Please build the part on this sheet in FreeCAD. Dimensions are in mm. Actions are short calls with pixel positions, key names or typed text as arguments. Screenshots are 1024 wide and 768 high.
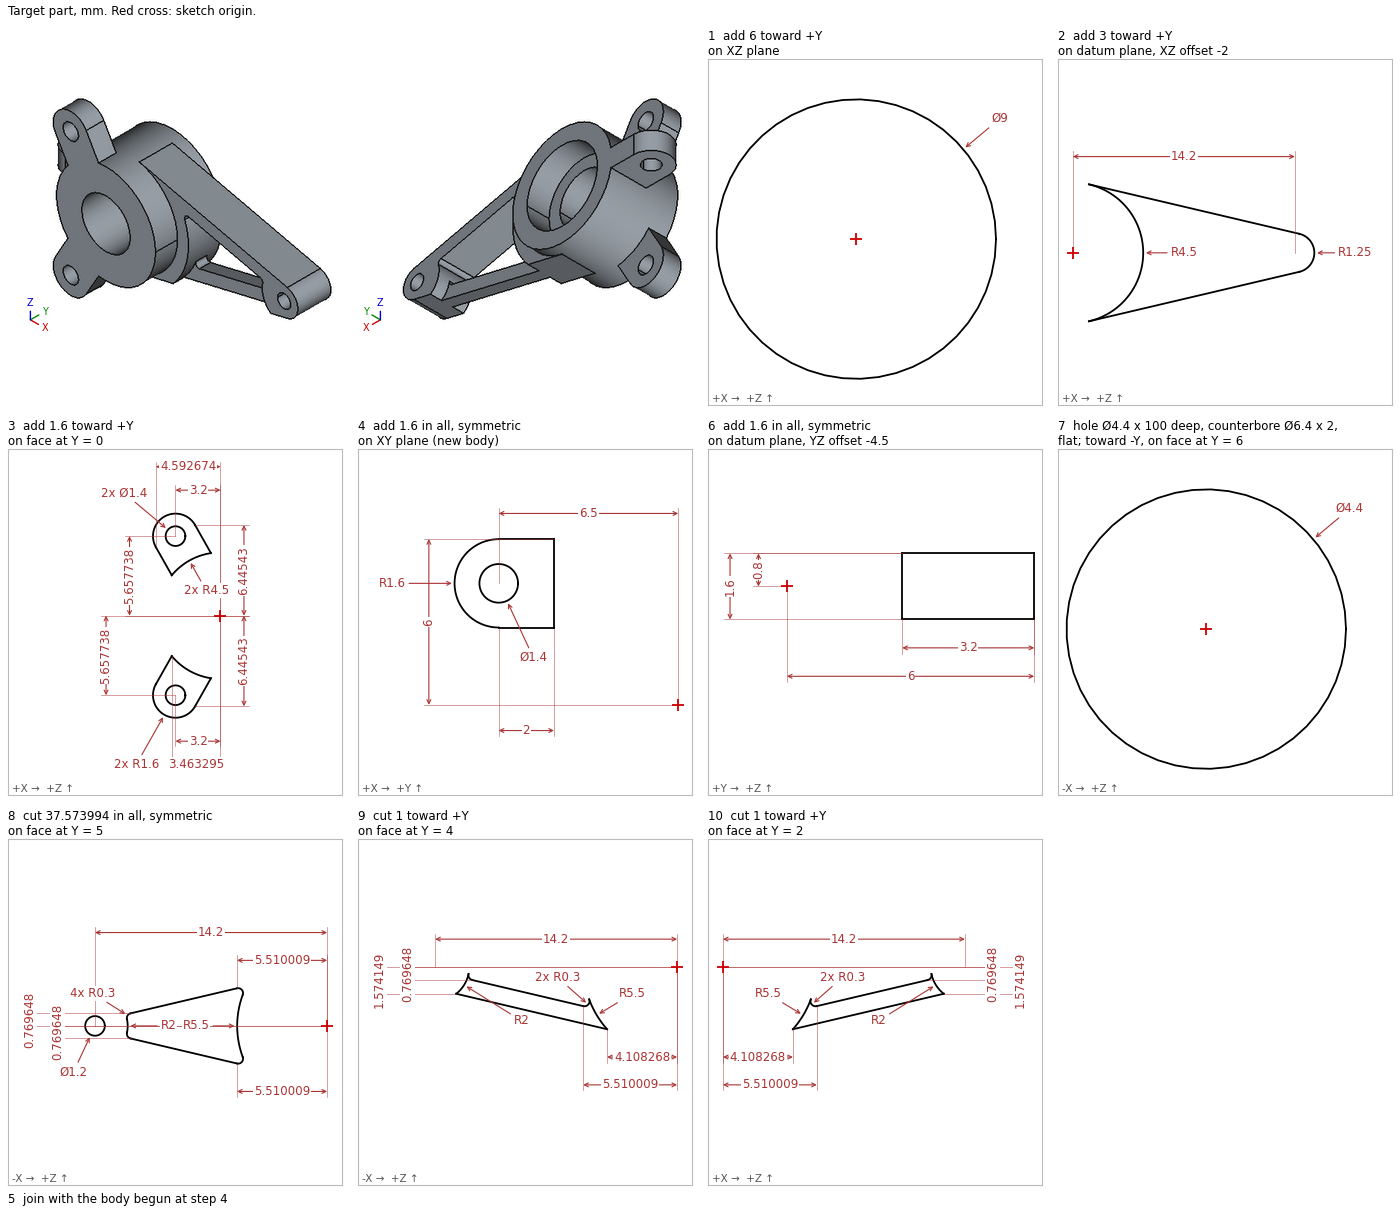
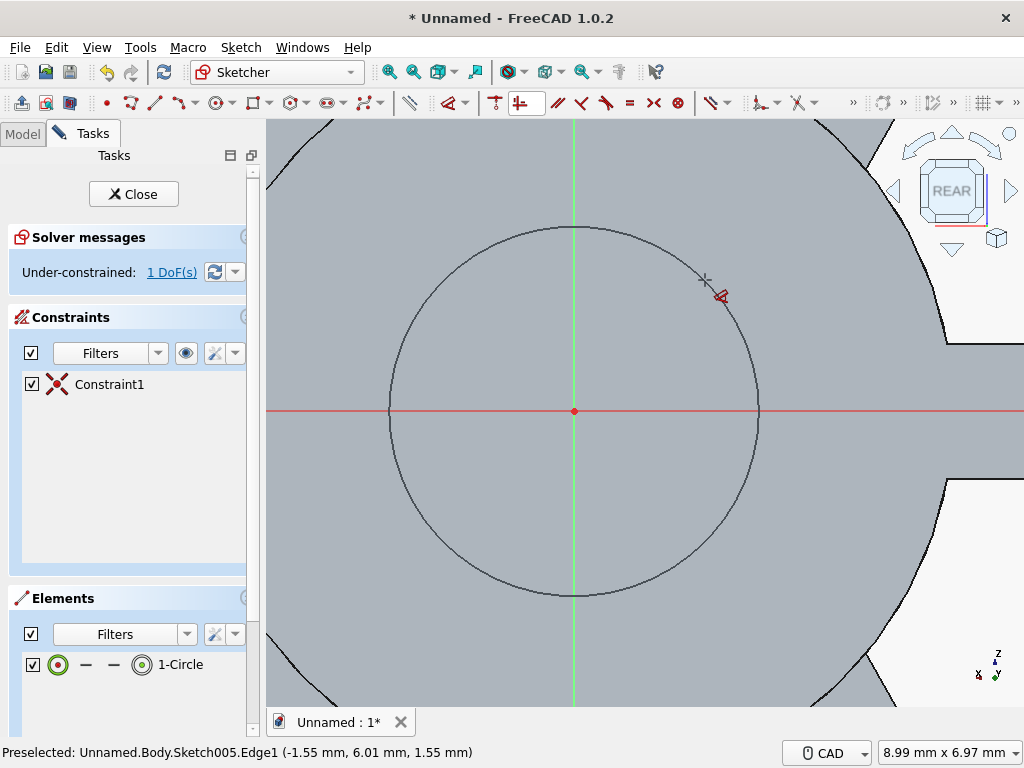
click(704, 280)
click(726, 257)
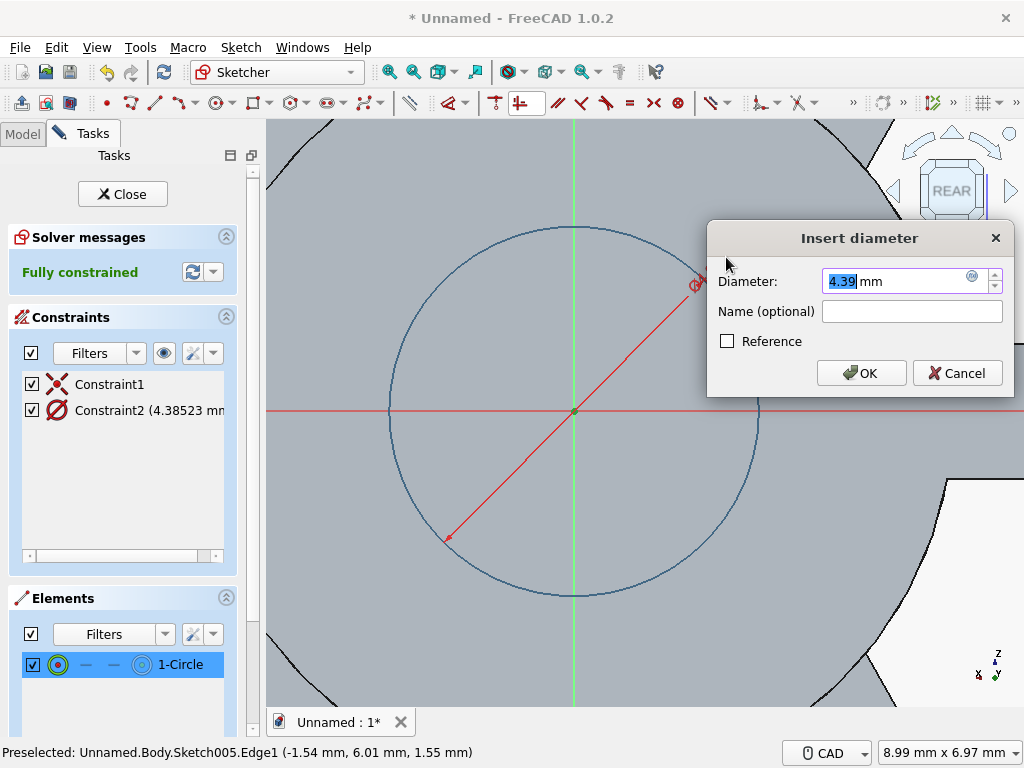
text(4.4)
key(Return)
key(Escape)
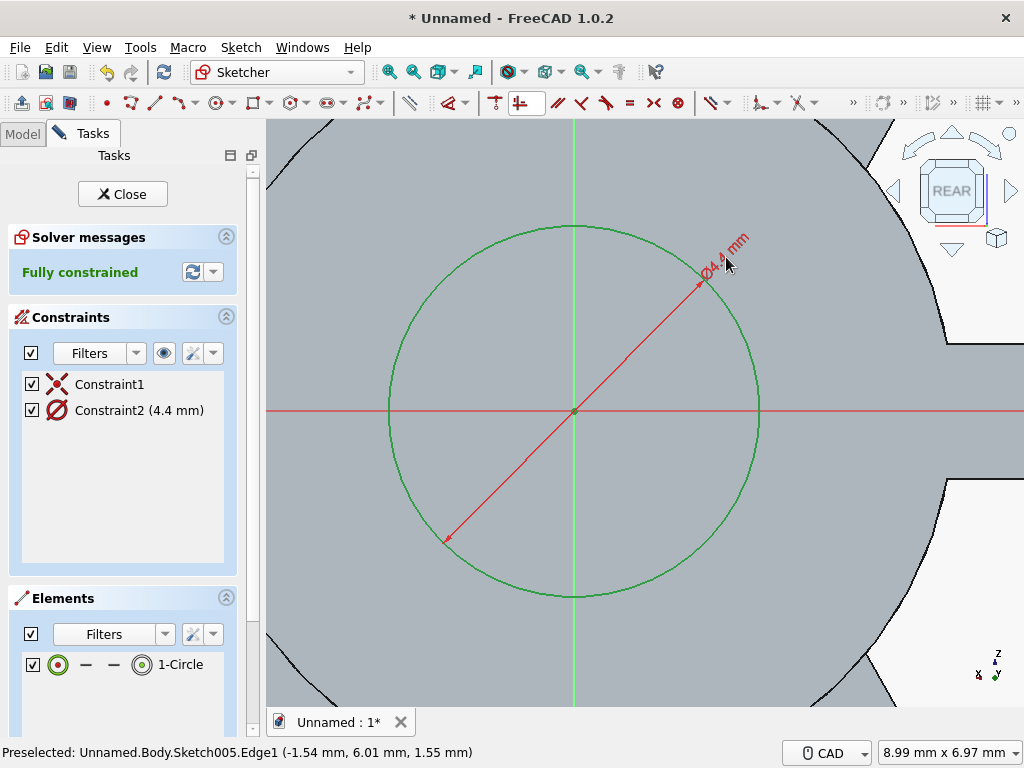
click(123, 194)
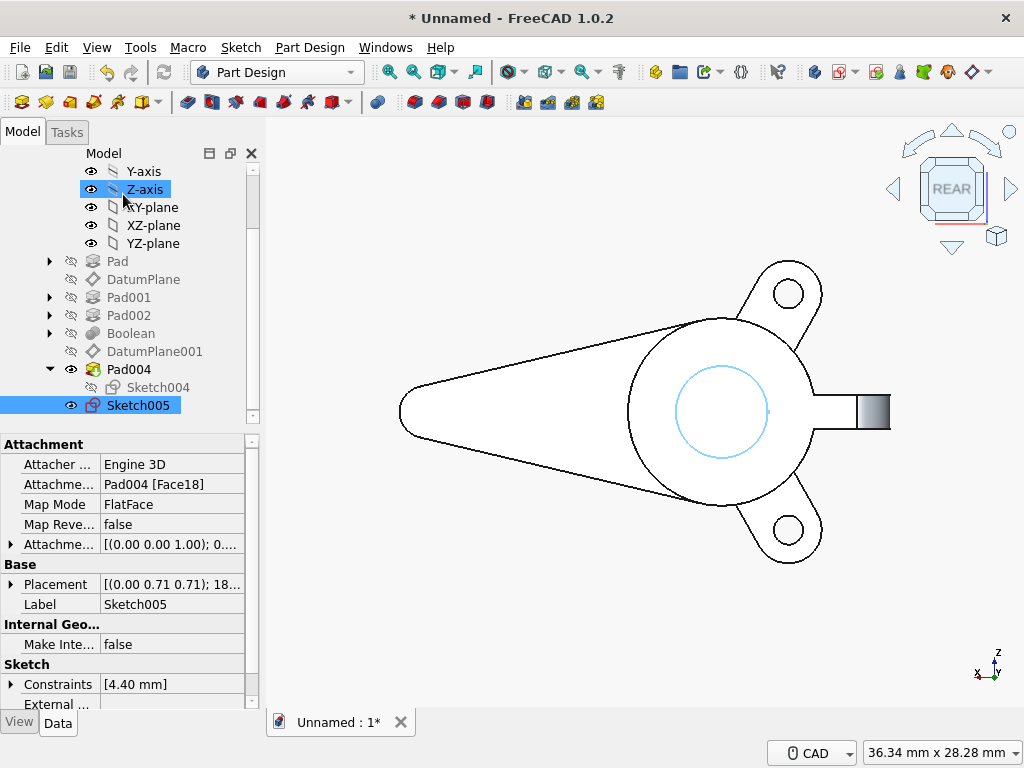
click(212, 102)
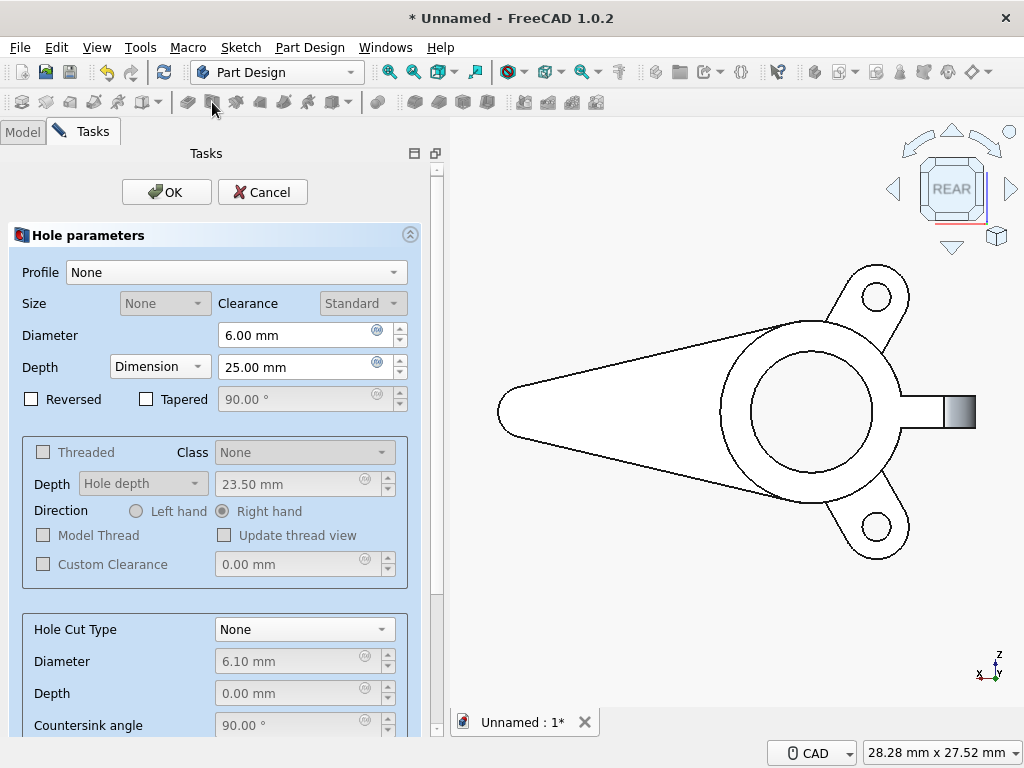
triple_click(305, 335)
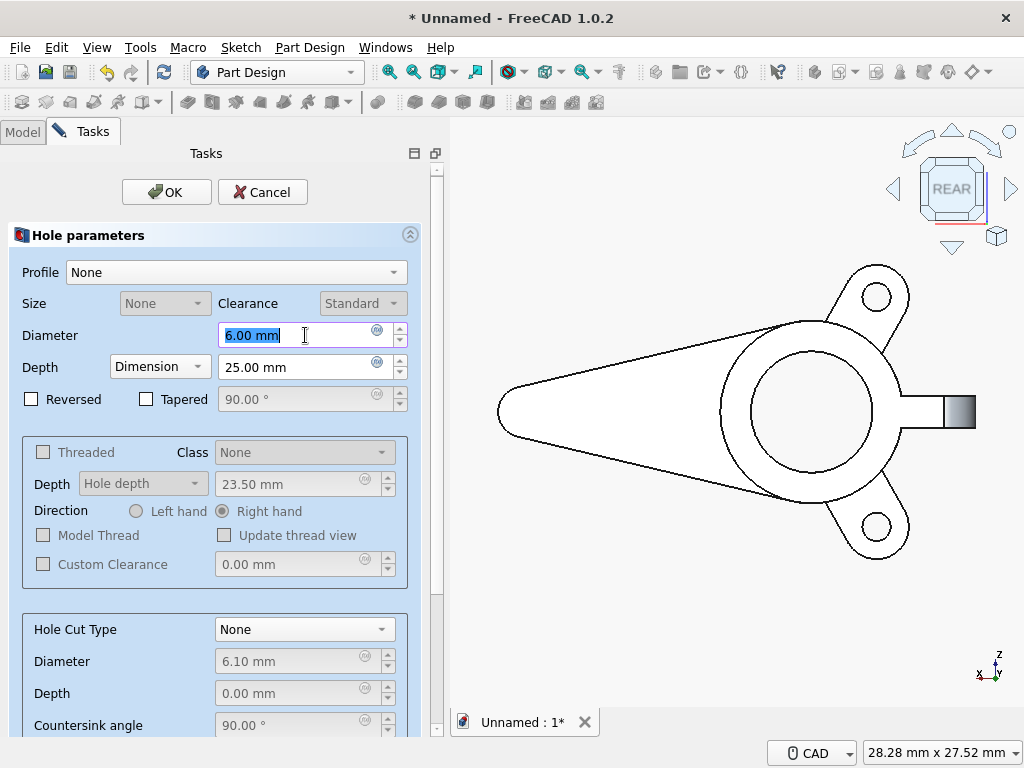
text(4.4)
key(Tab)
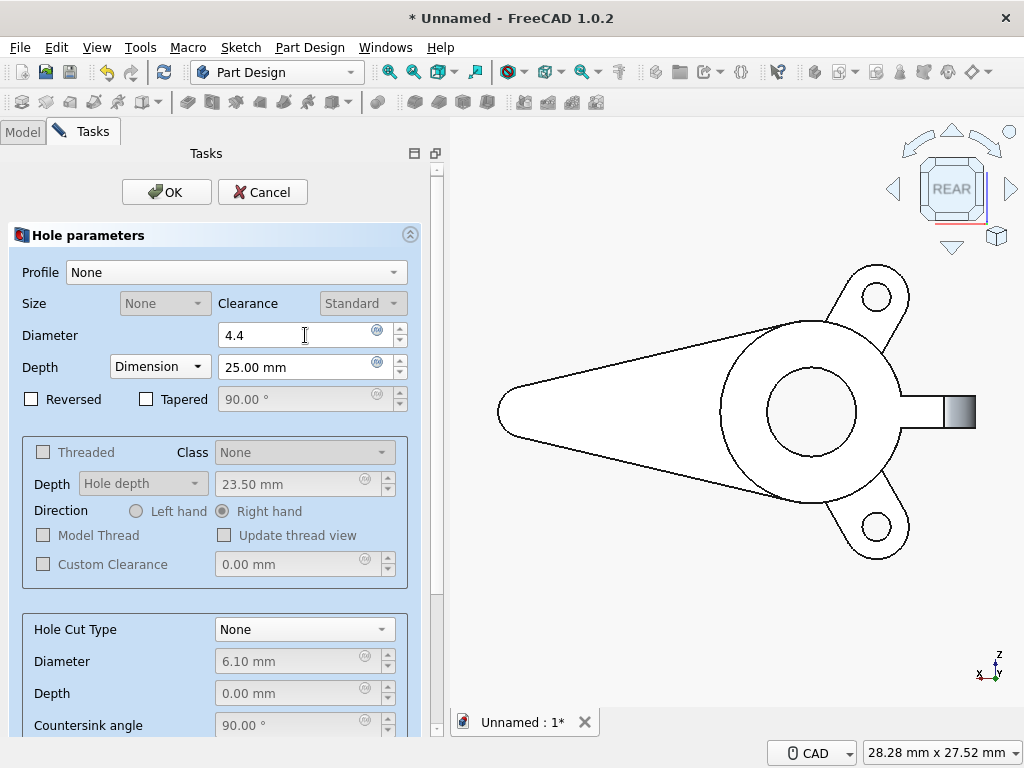
triple_click(305, 367)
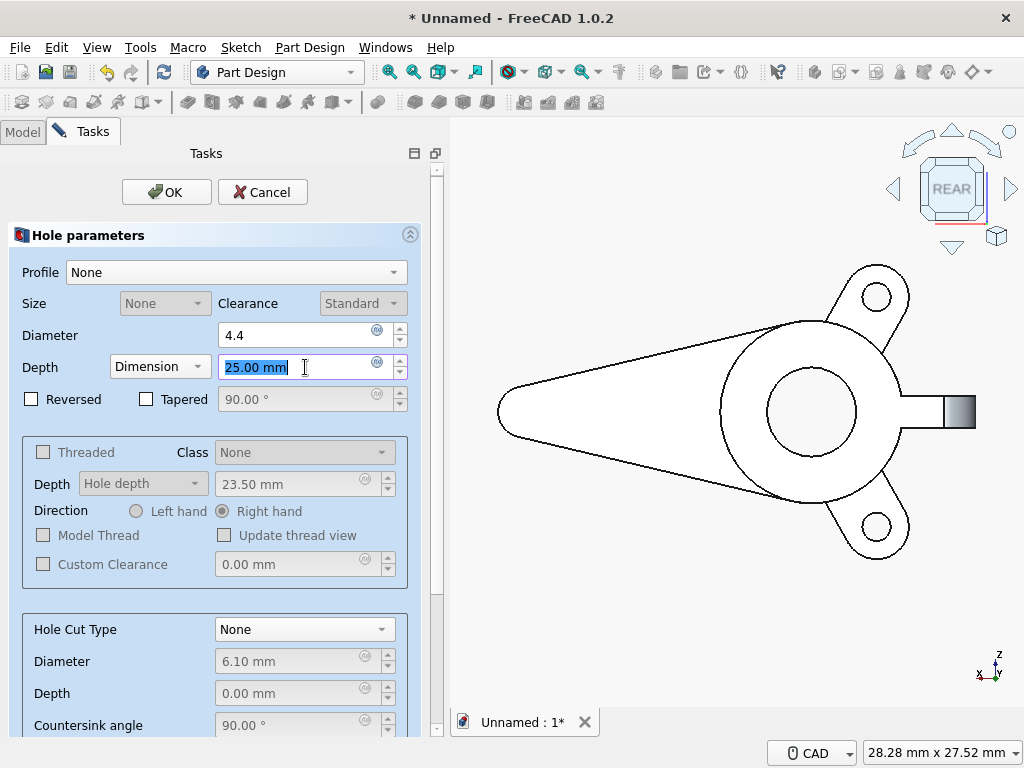
text(100)
key(Tab)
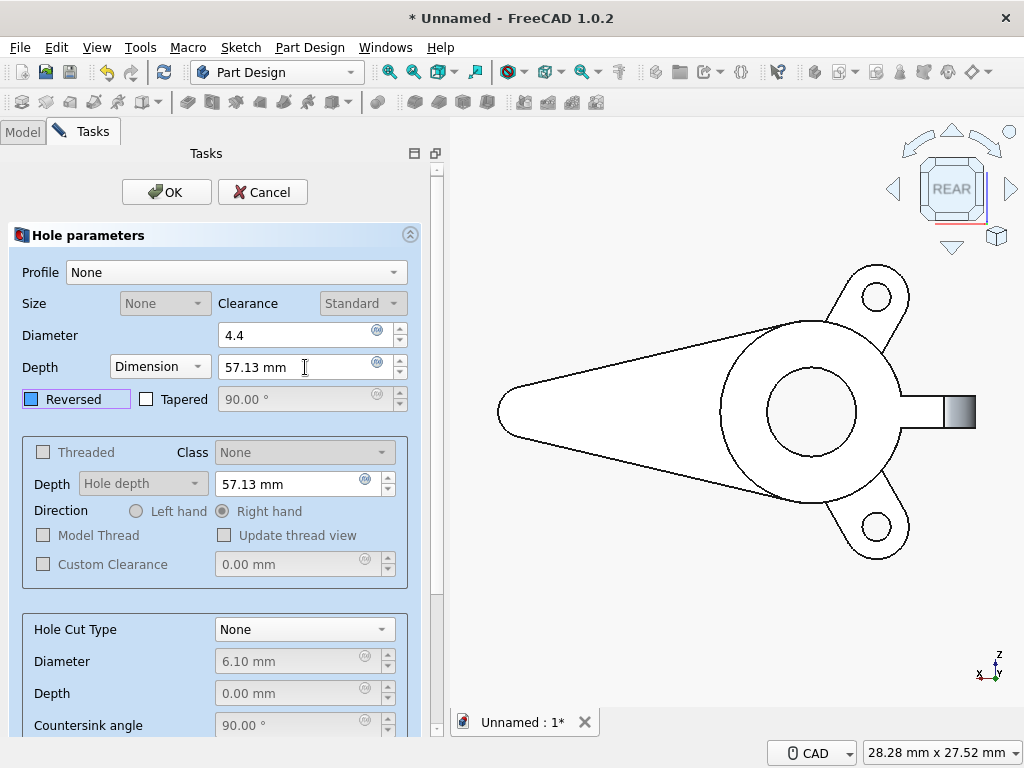
click(306, 630)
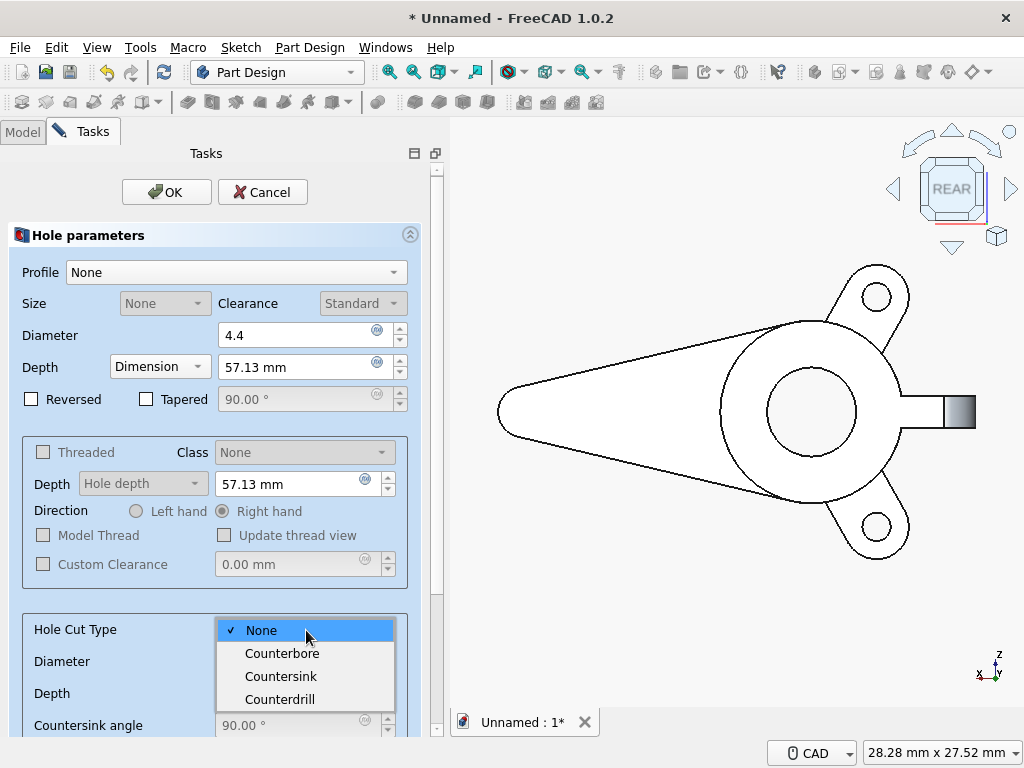
click(304, 654)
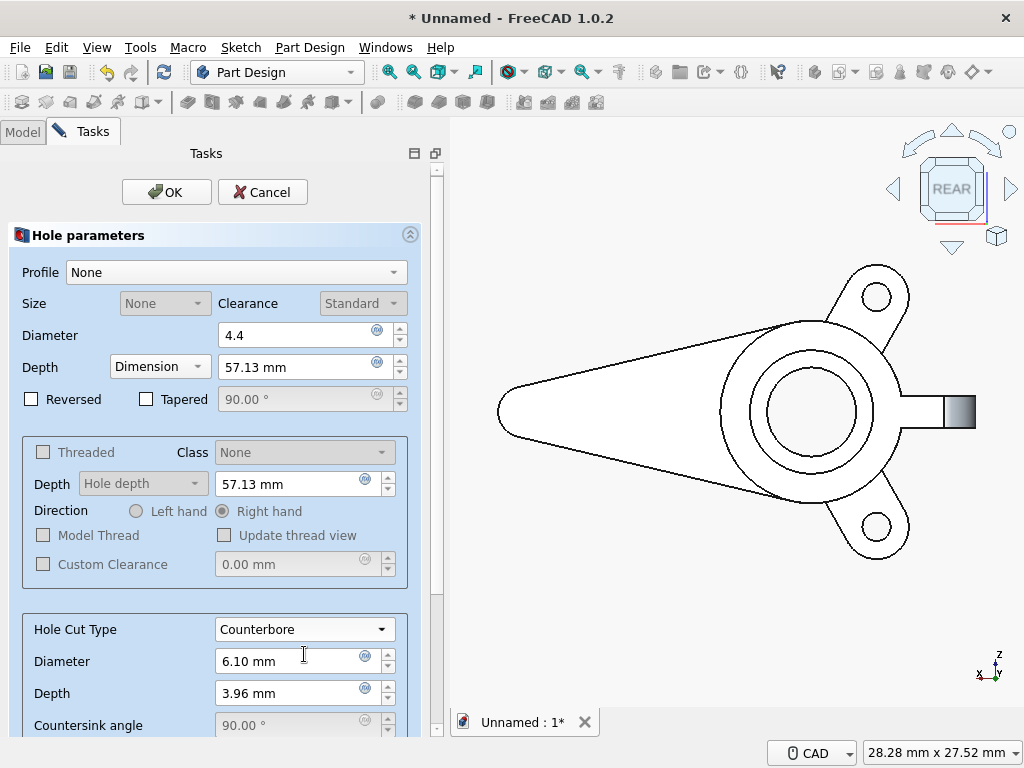
triple_click(298, 661)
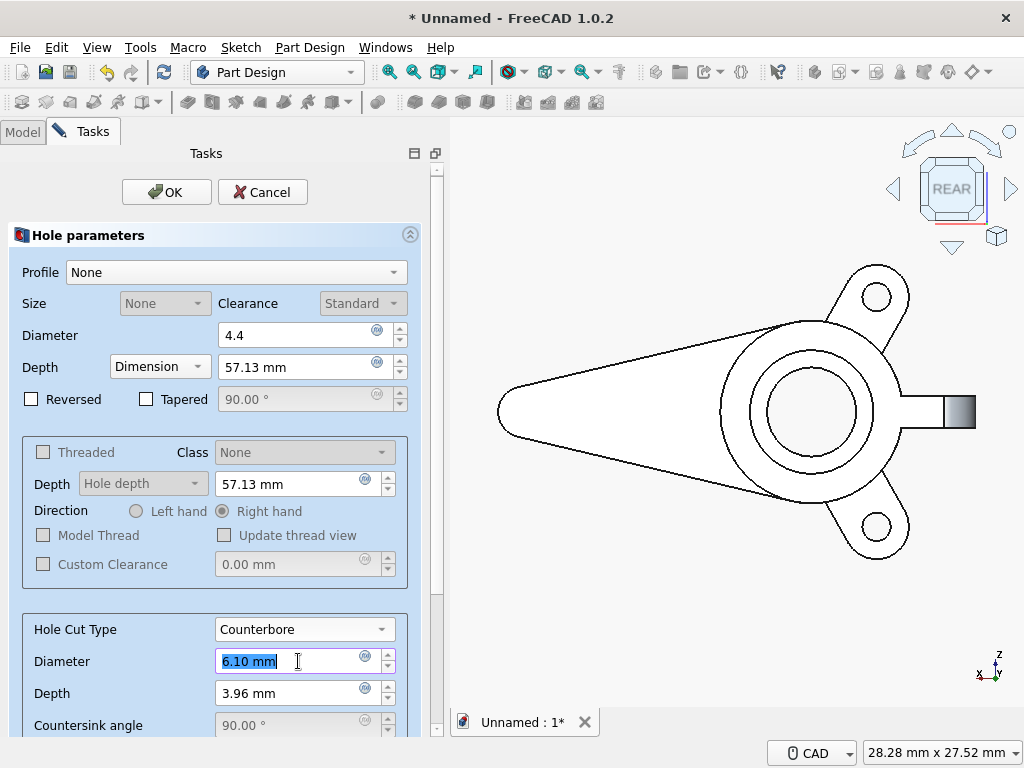
text(6.4)
key(Tab)